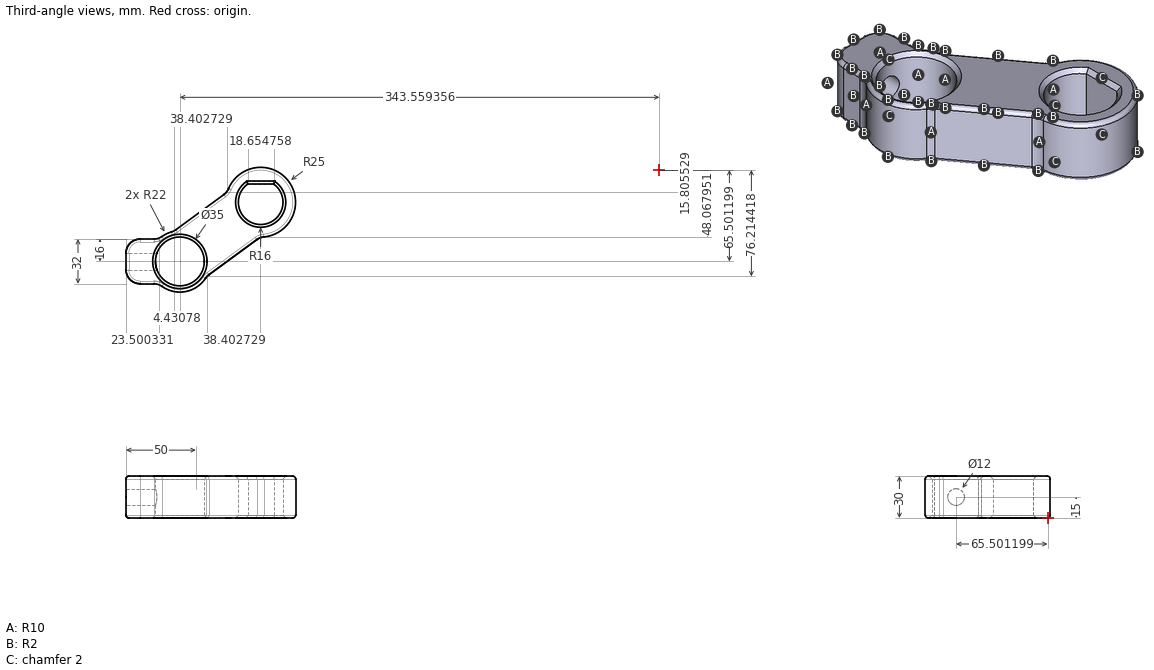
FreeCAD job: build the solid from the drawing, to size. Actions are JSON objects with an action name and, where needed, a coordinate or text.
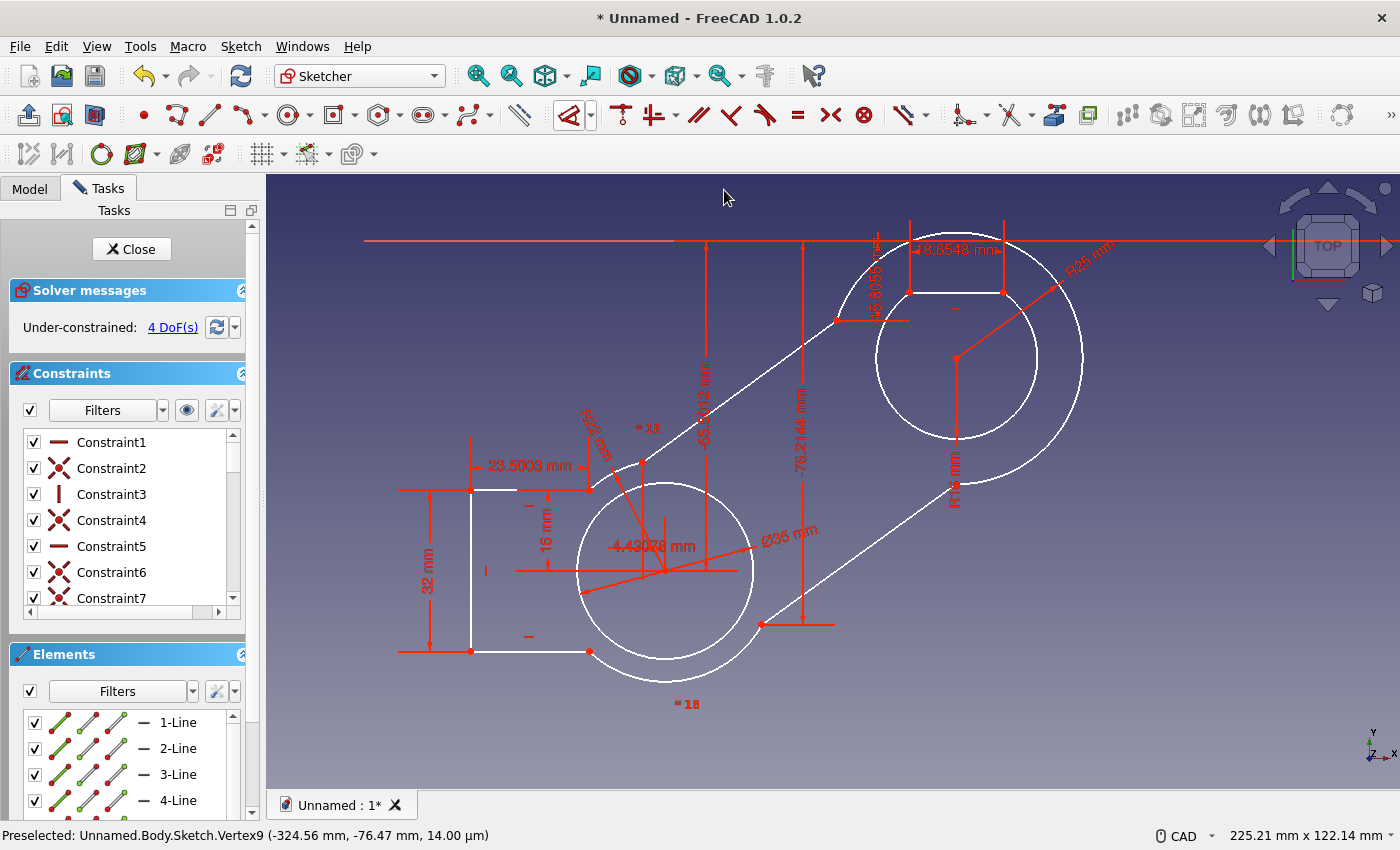
{"action": "left_click", "coordinate": [956, 484]}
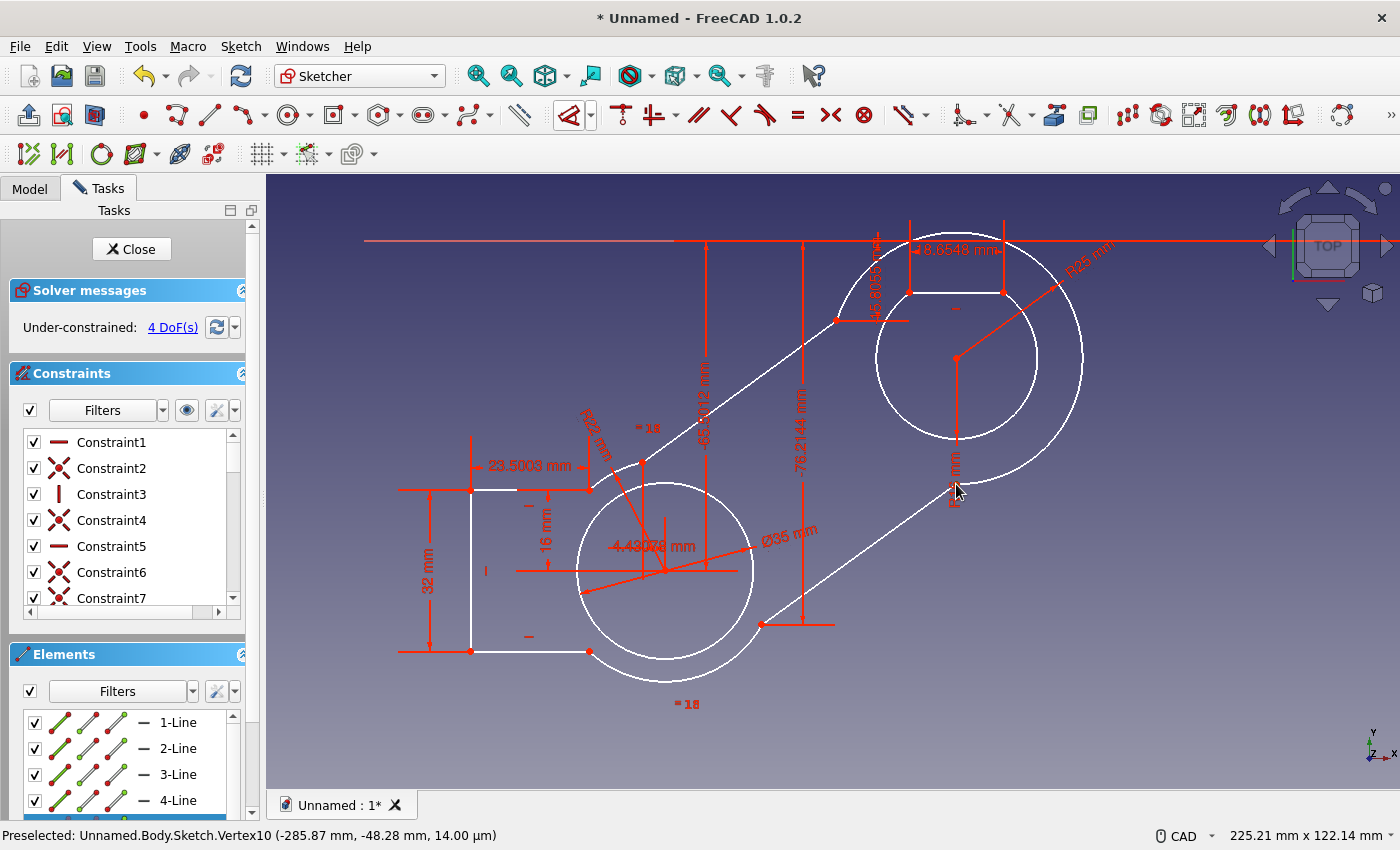
{"action": "key", "text": "i"}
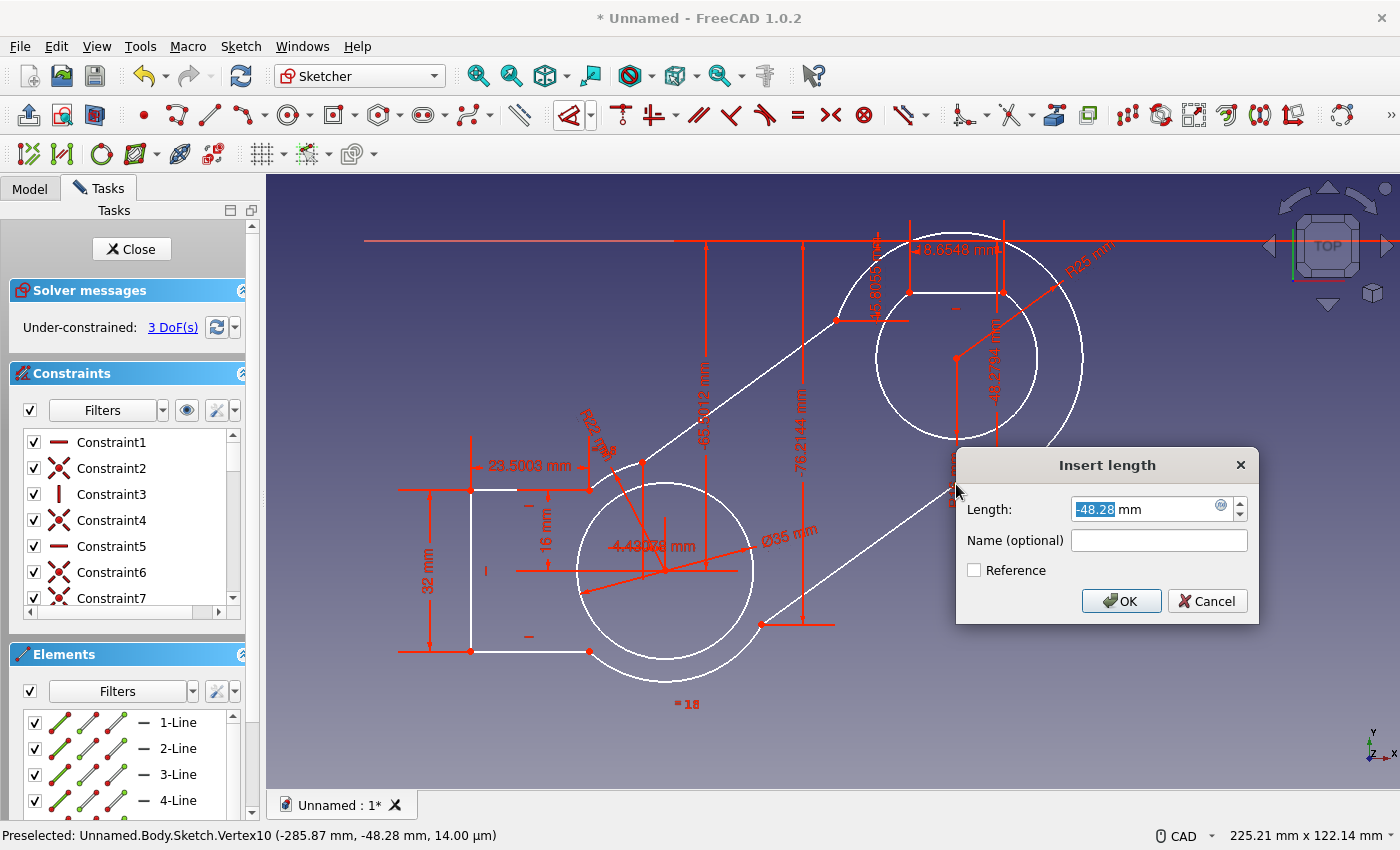
{"action": "type", "text": "-48.067951"}
{"action": "key", "text": "Return"}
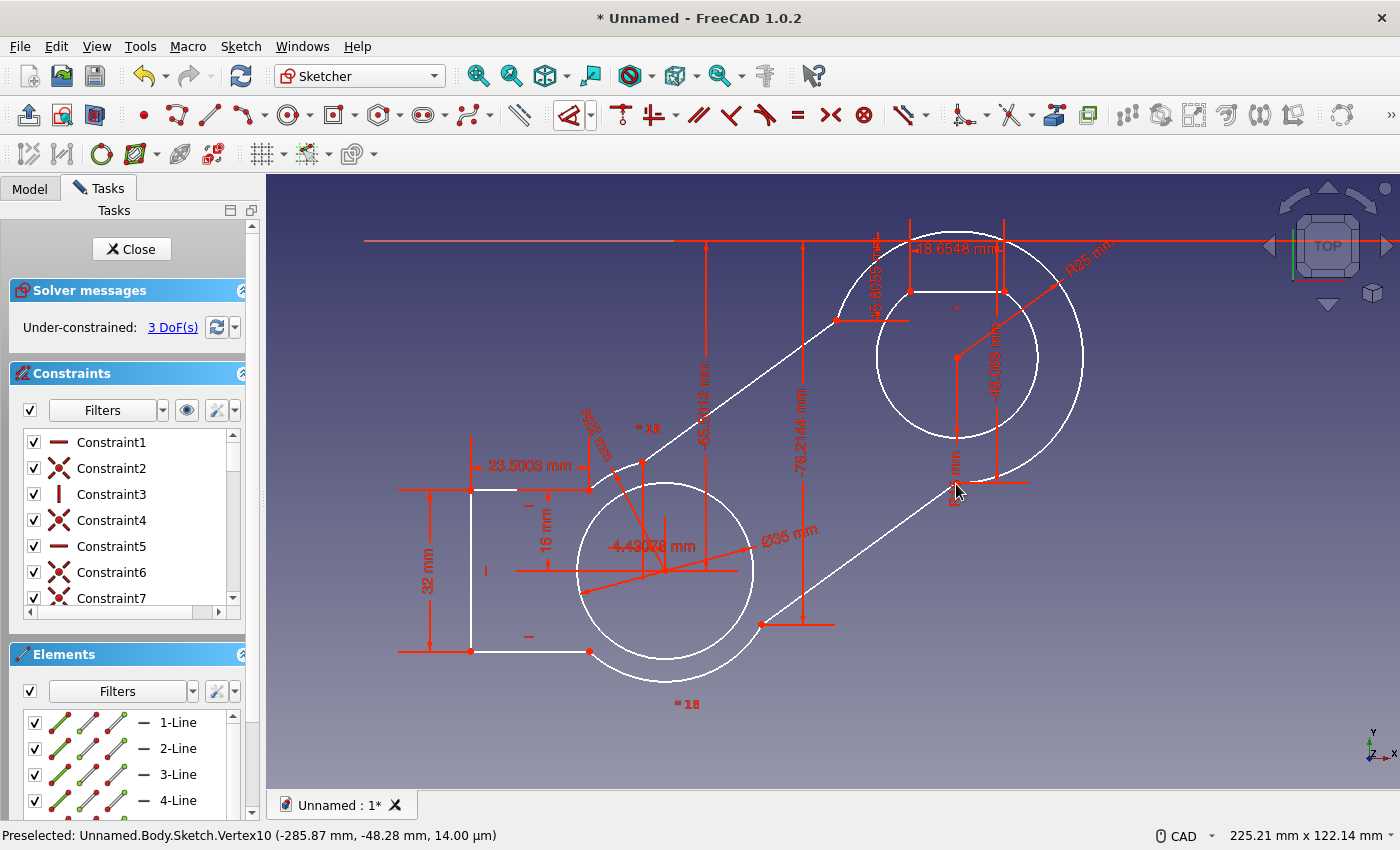
{"action": "left_click", "coordinate": [779, 363]}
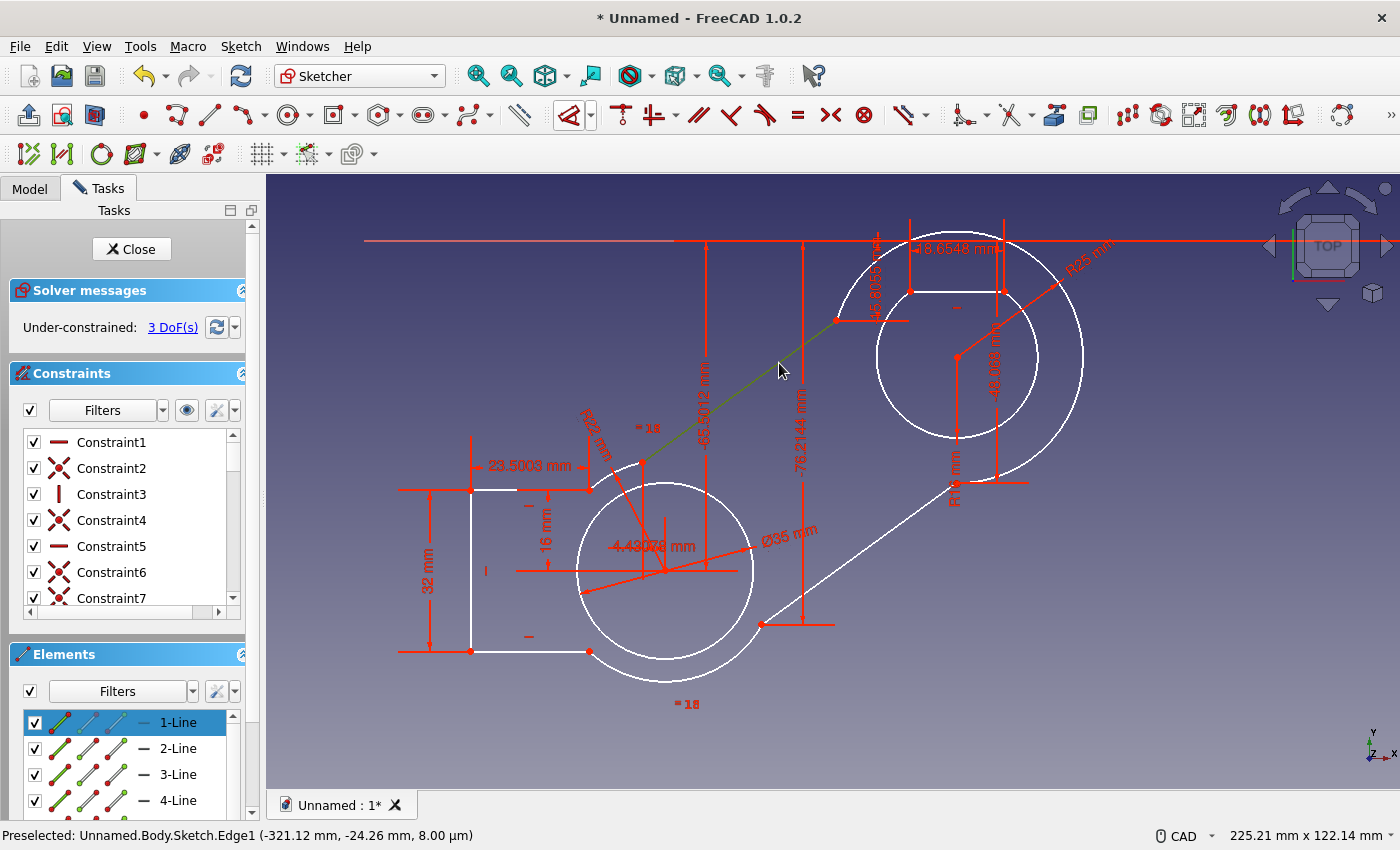
{"action": "left_click", "coordinate": [590, 116]}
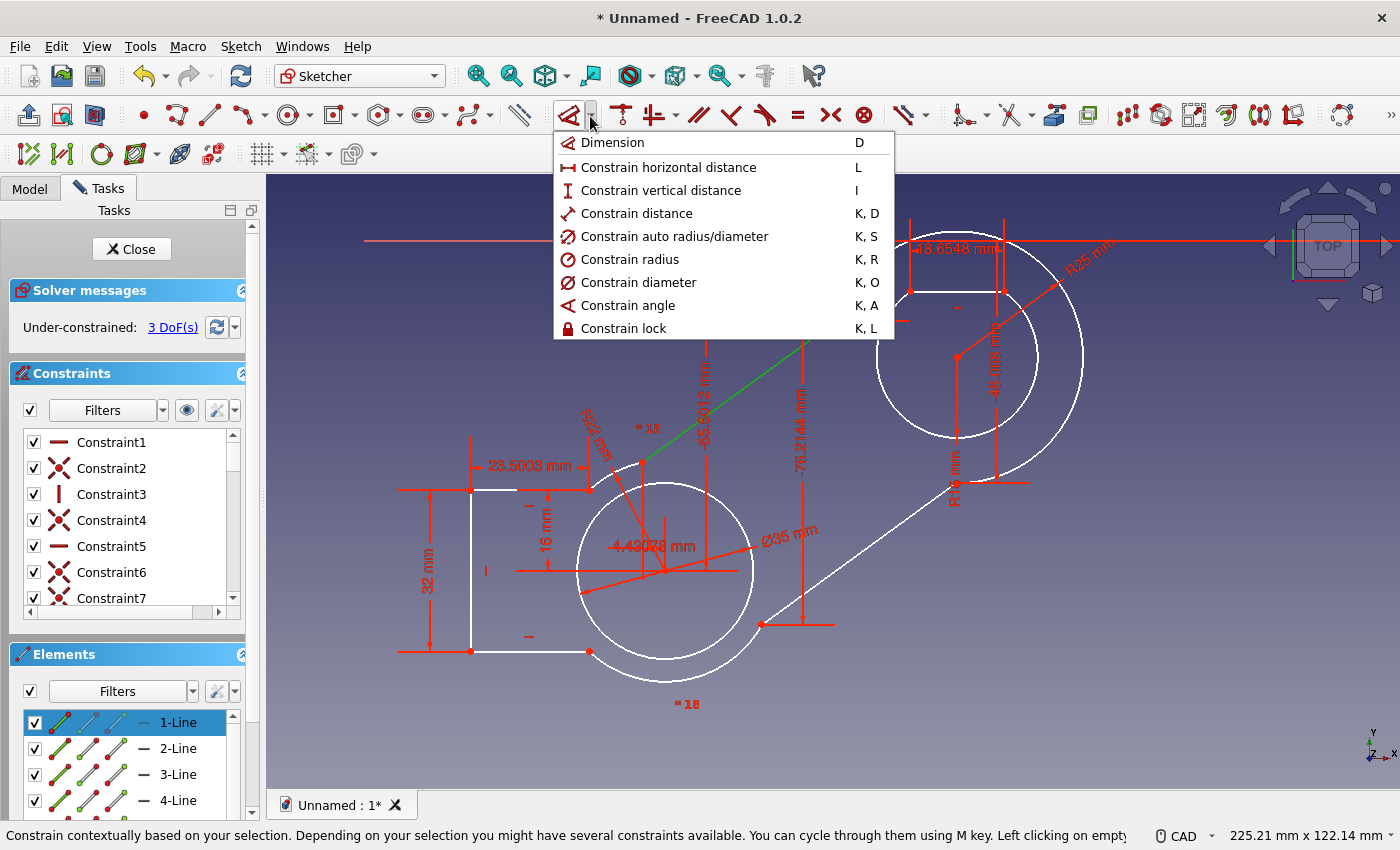
{"action": "left_click", "coordinate": [724, 168]}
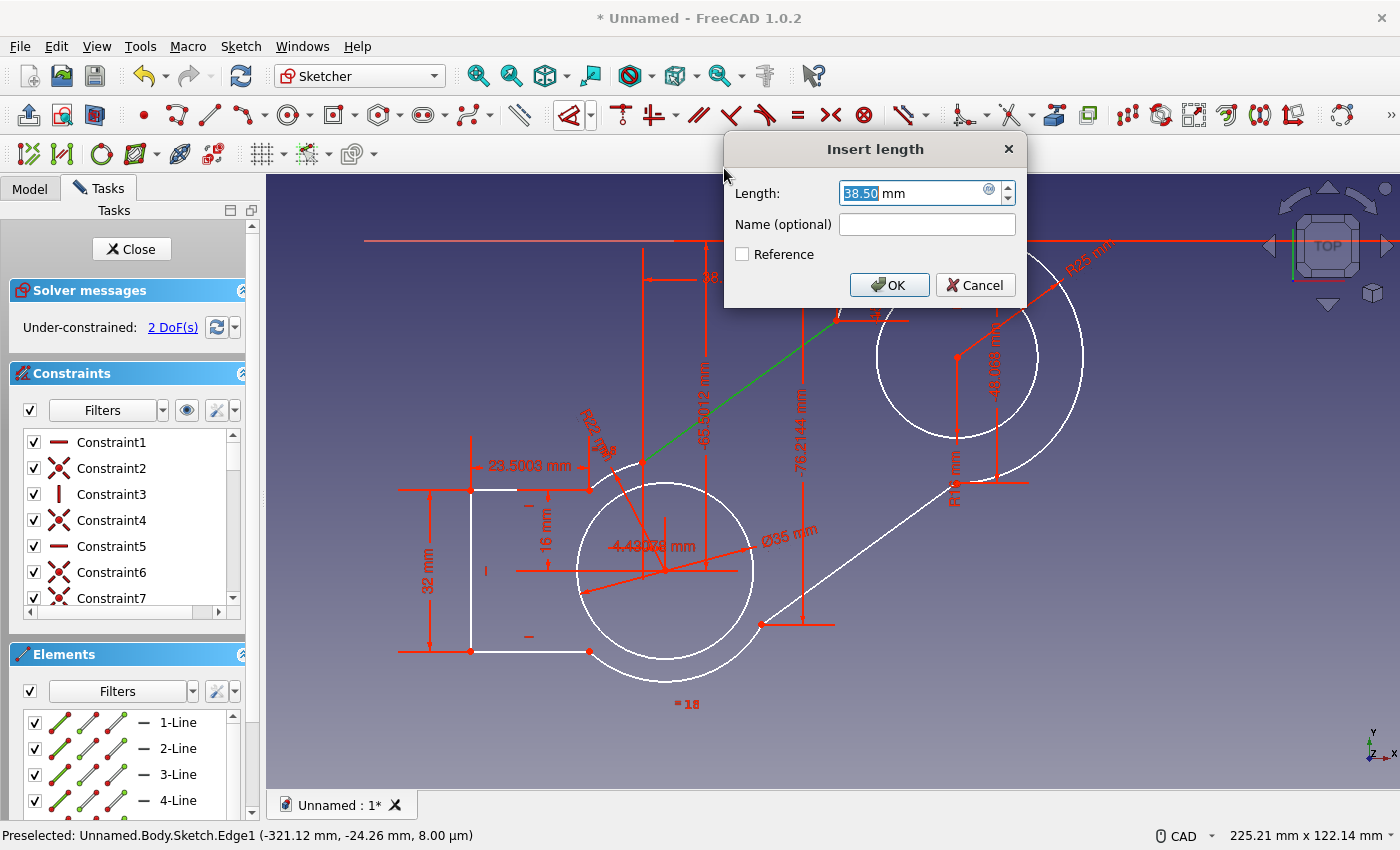
{"action": "type", "text": "38.402729"}
{"action": "key", "text": "Return"}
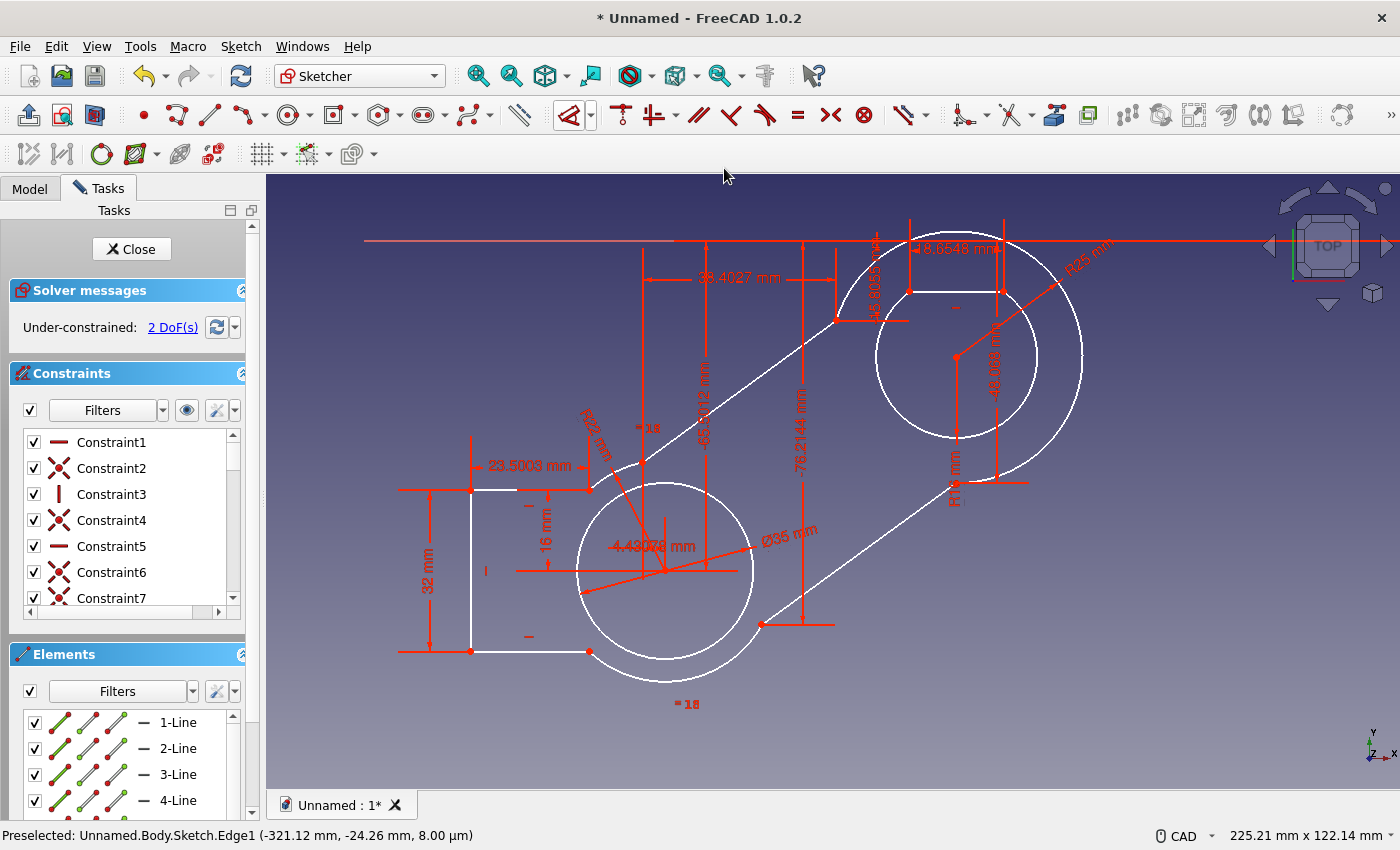
{"action": "left_click", "coordinate": [820, 582]}